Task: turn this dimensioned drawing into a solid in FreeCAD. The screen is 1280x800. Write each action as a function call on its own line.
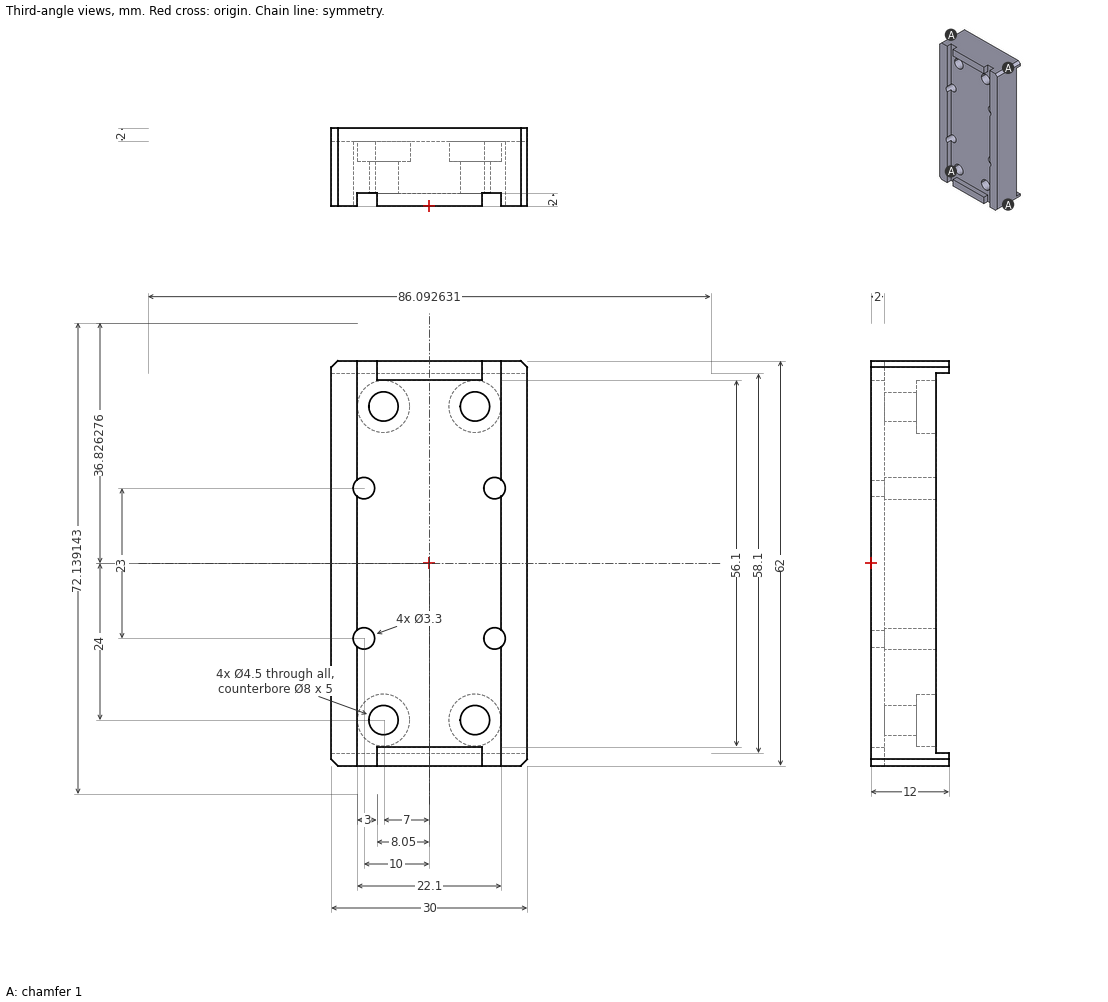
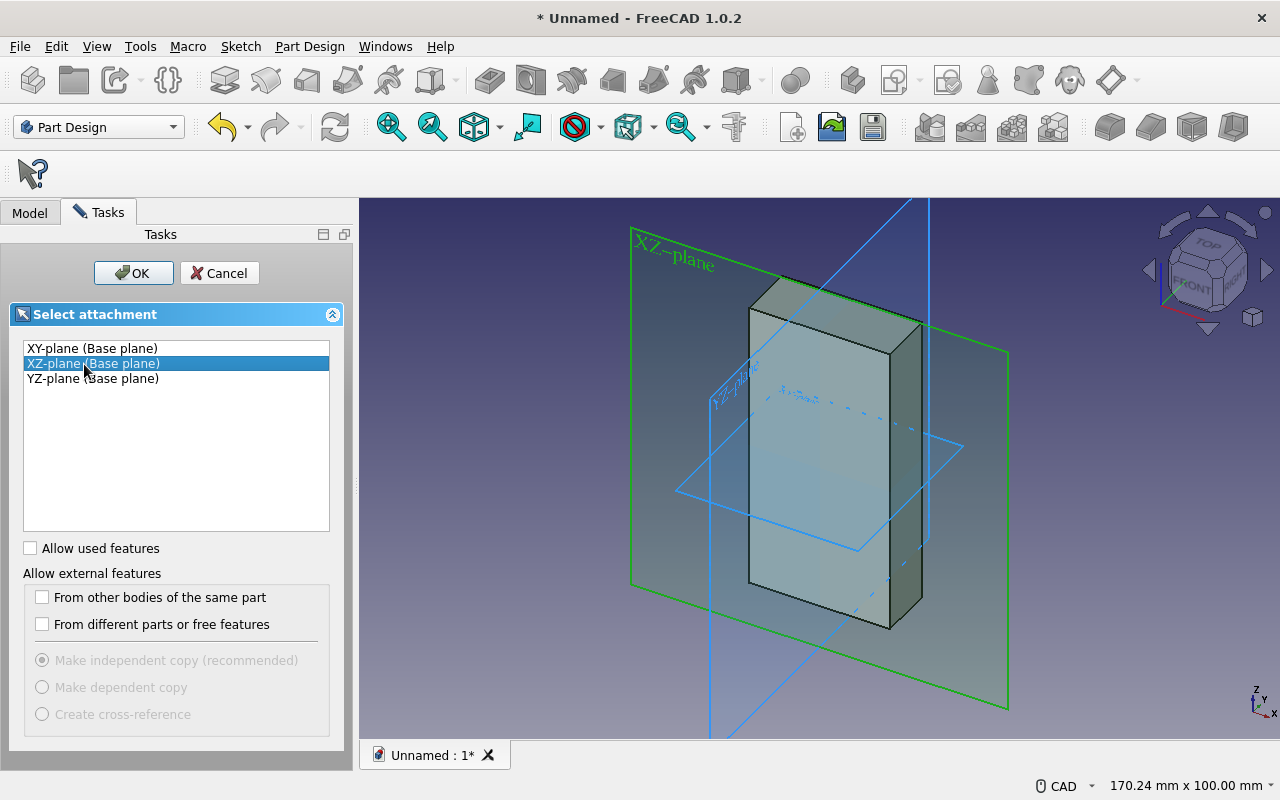
click(134, 273)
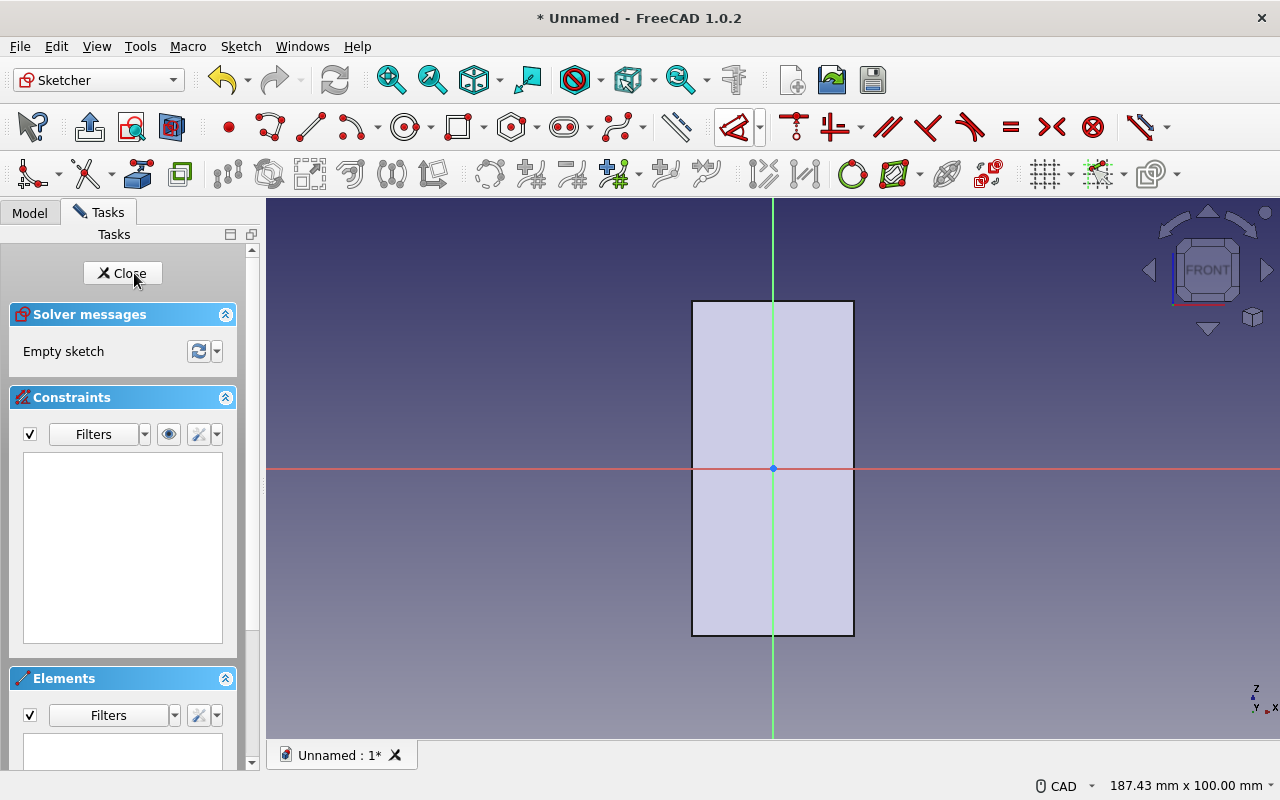
click(484, 128)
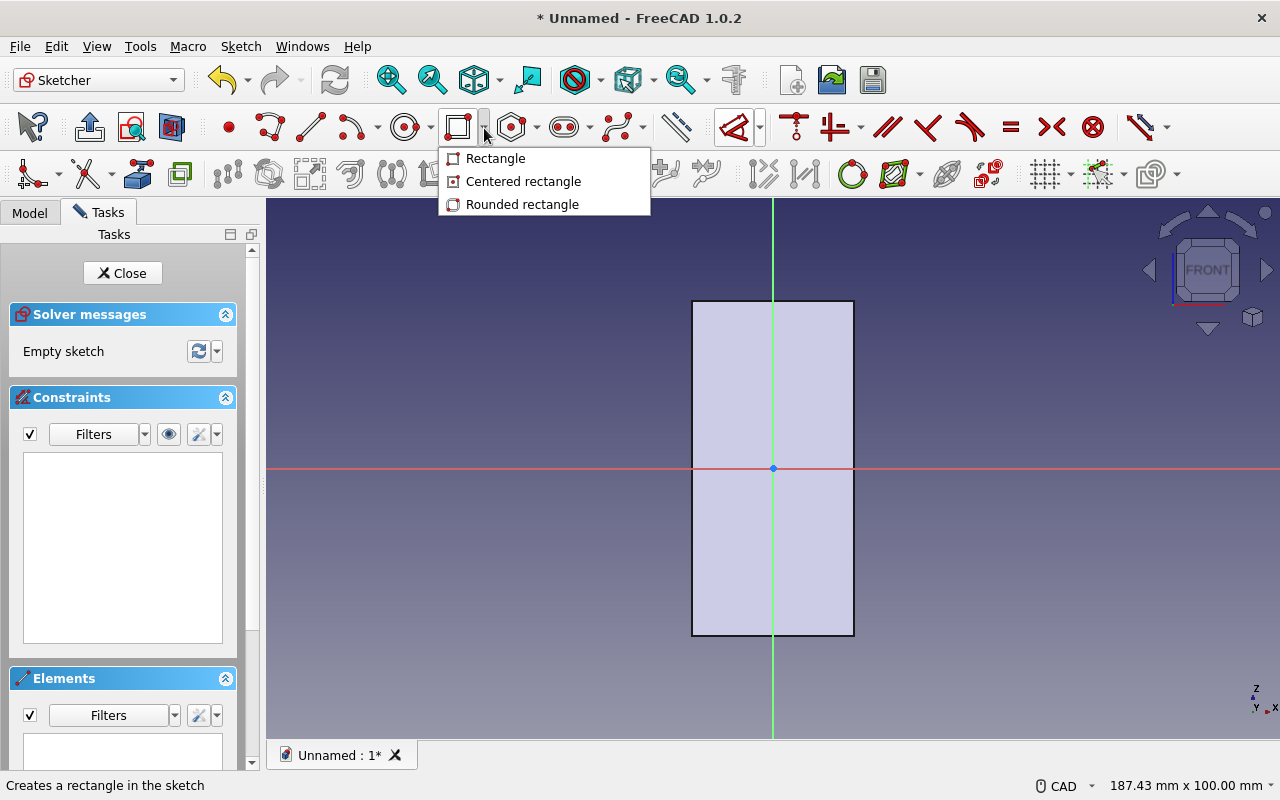
click(544, 182)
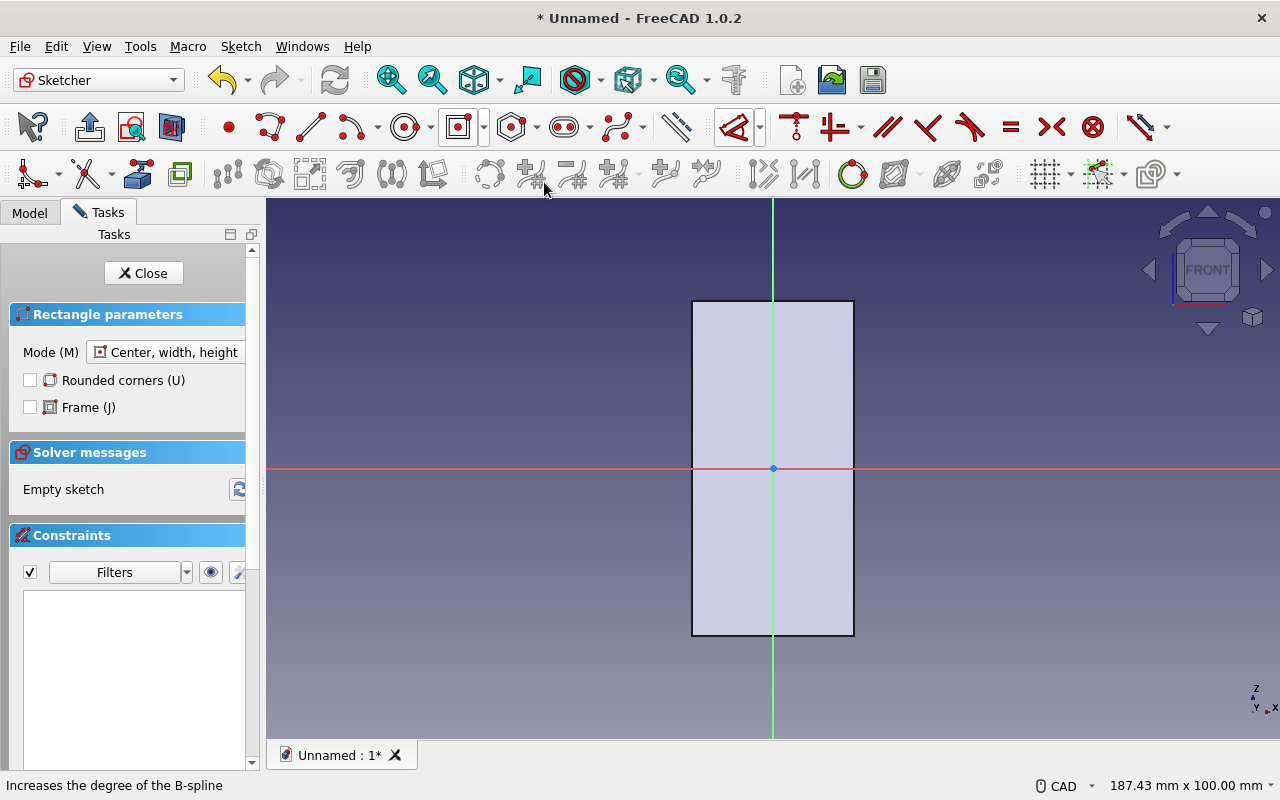
click(773, 468)
click(833, 317)
key(Escape)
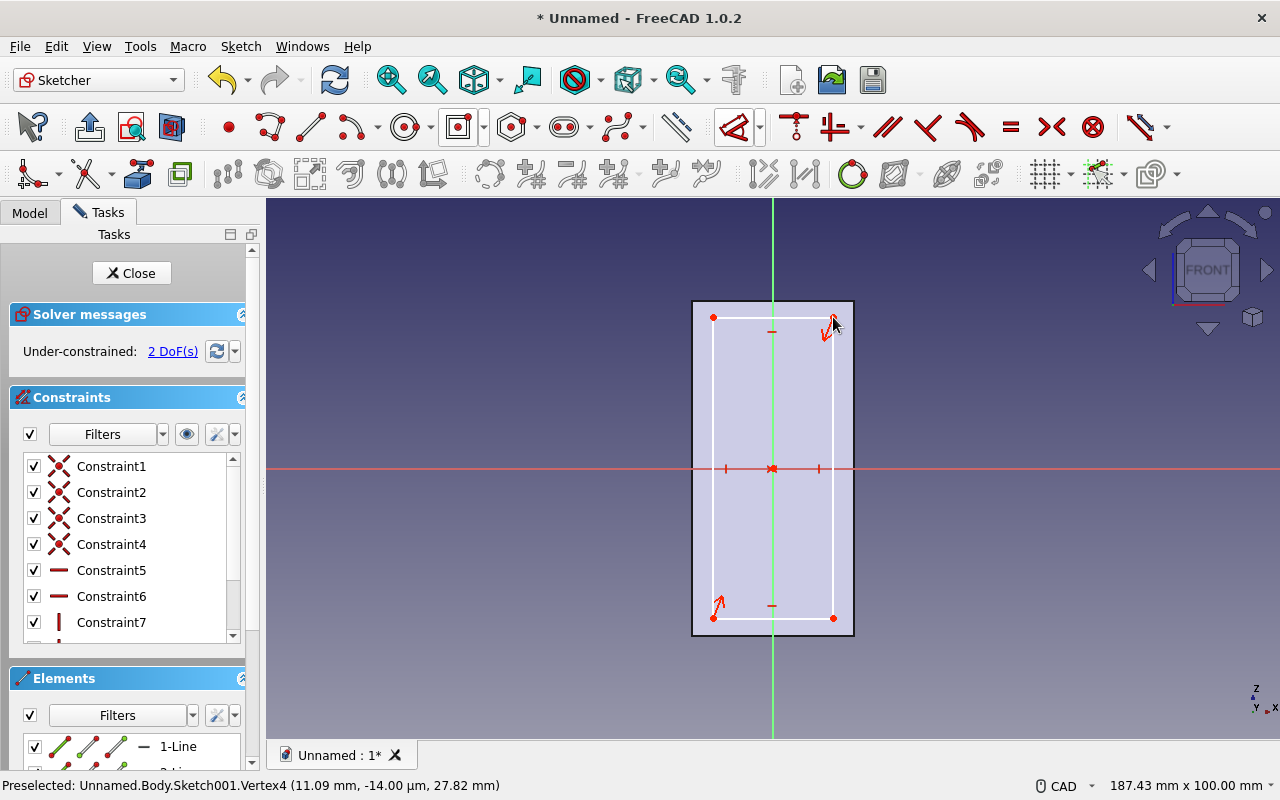
click(749, 619)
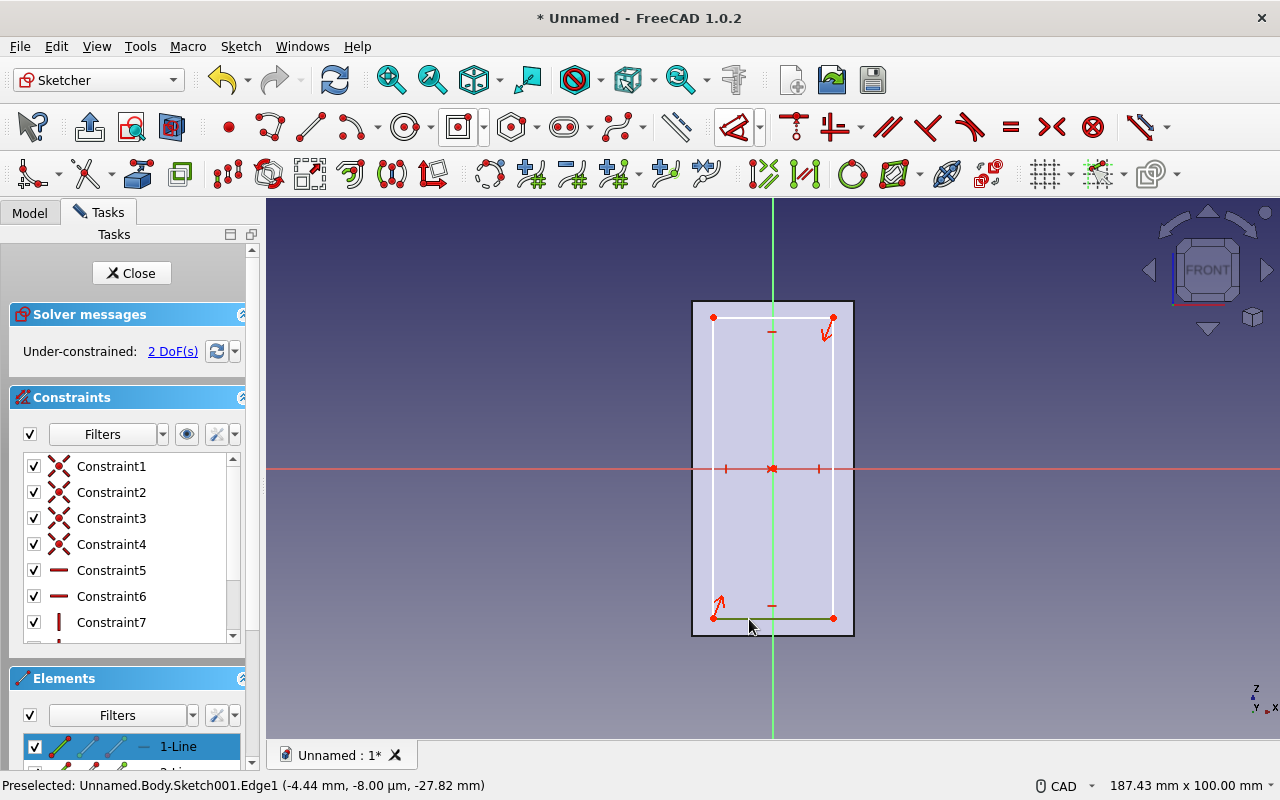
click(760, 128)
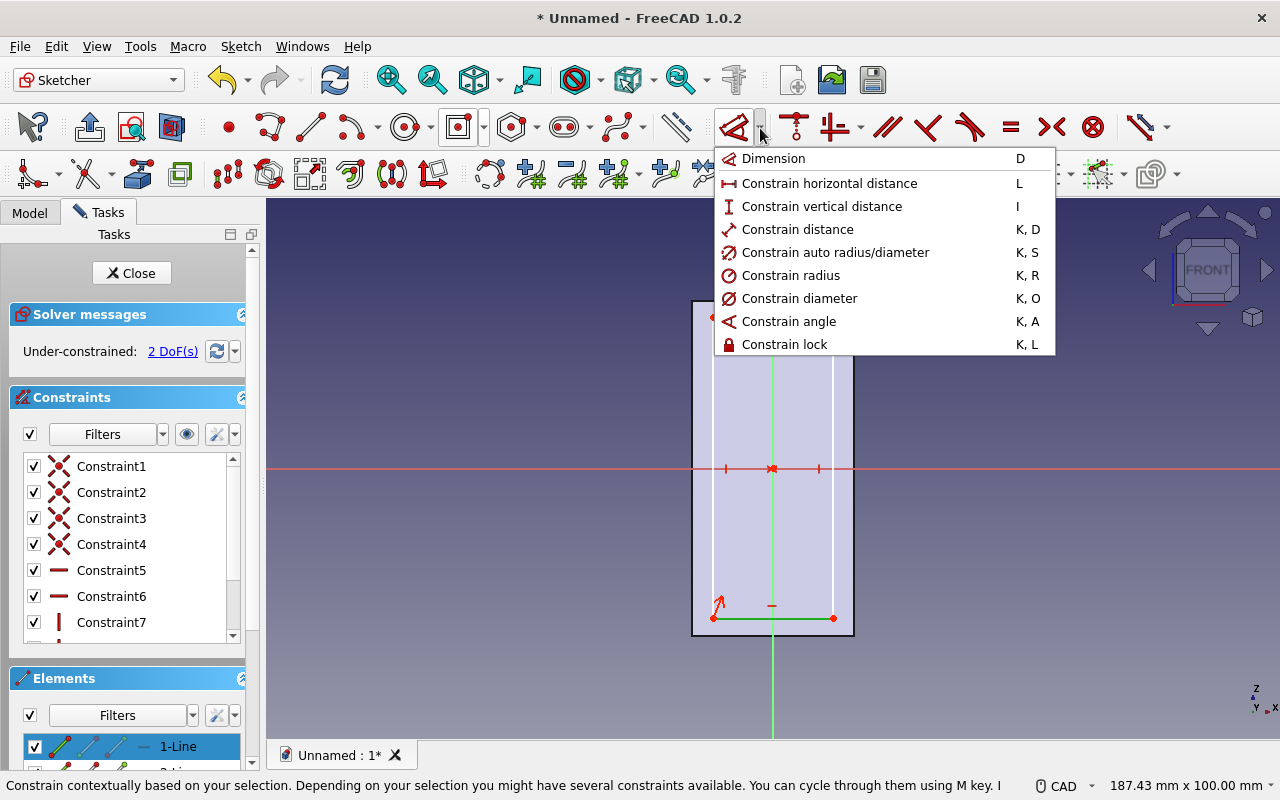
click(885, 184)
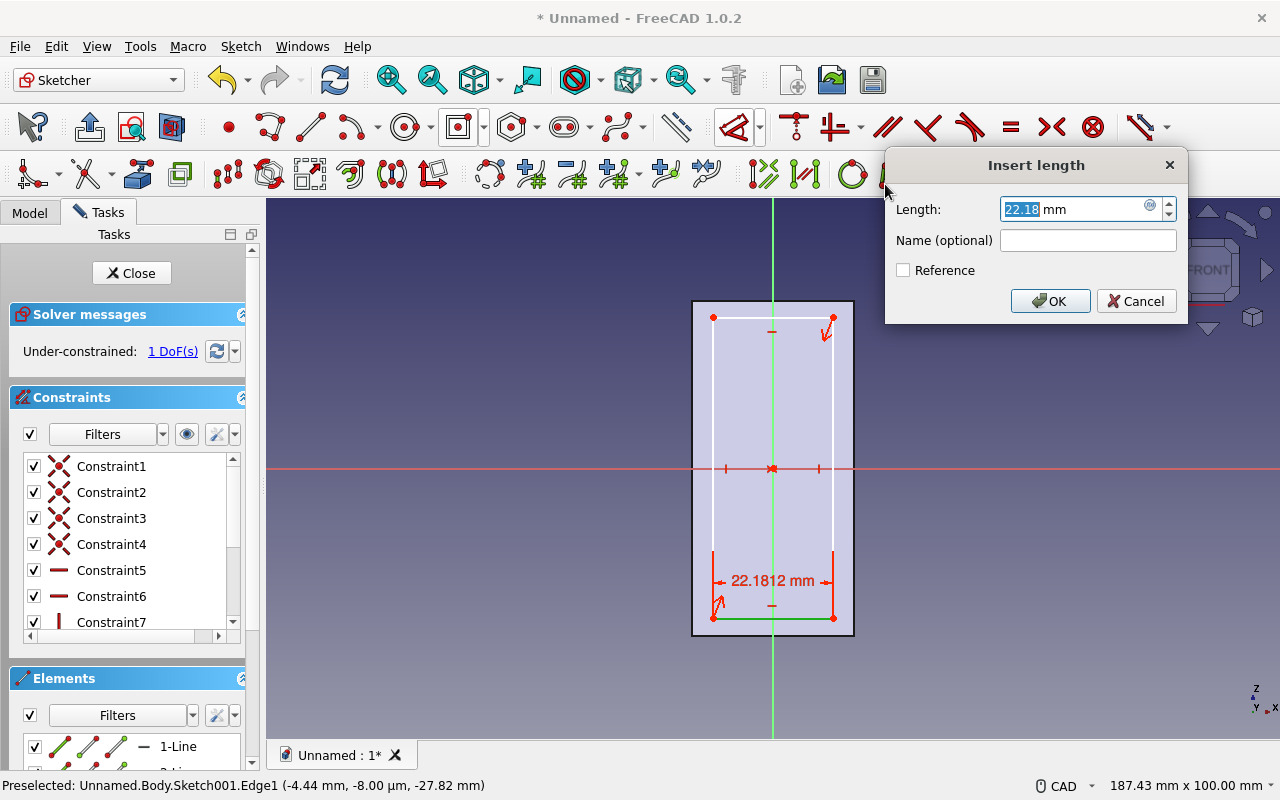
text(22.1)
key(Return)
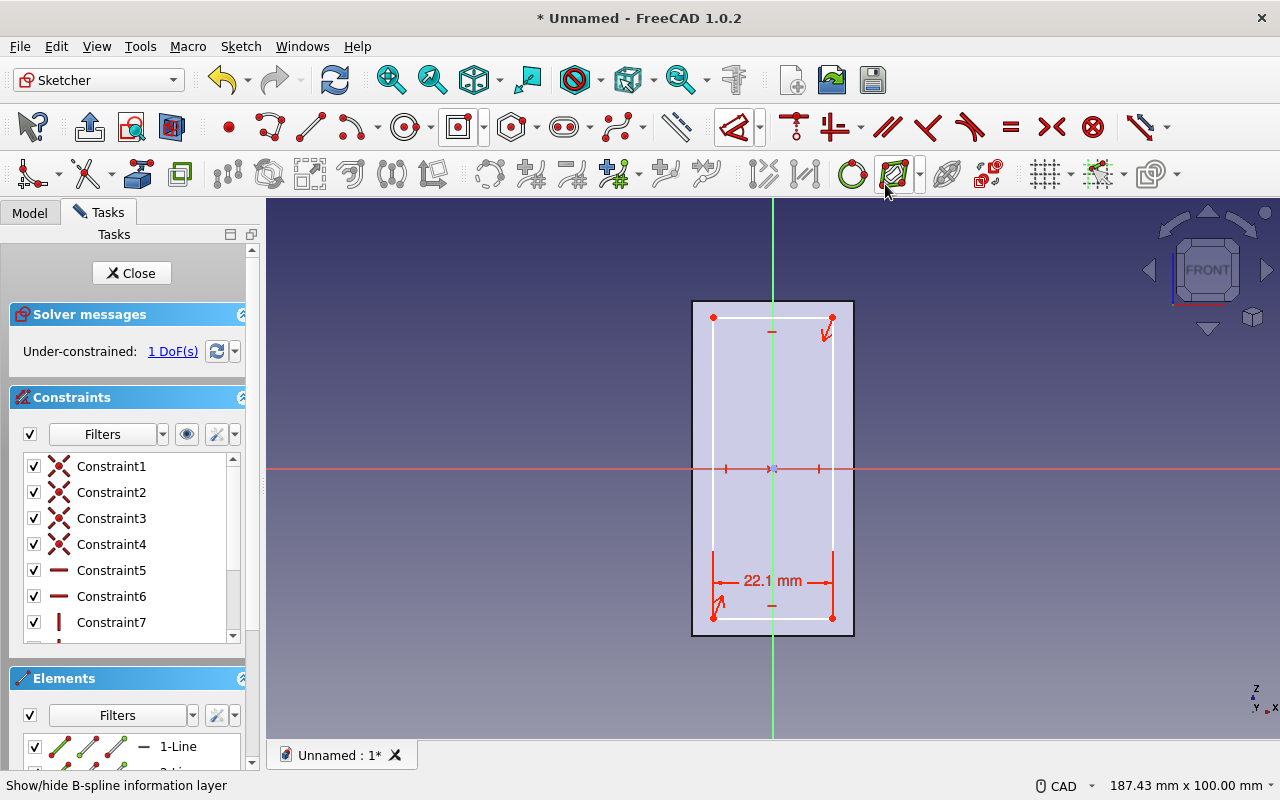
click(833, 529)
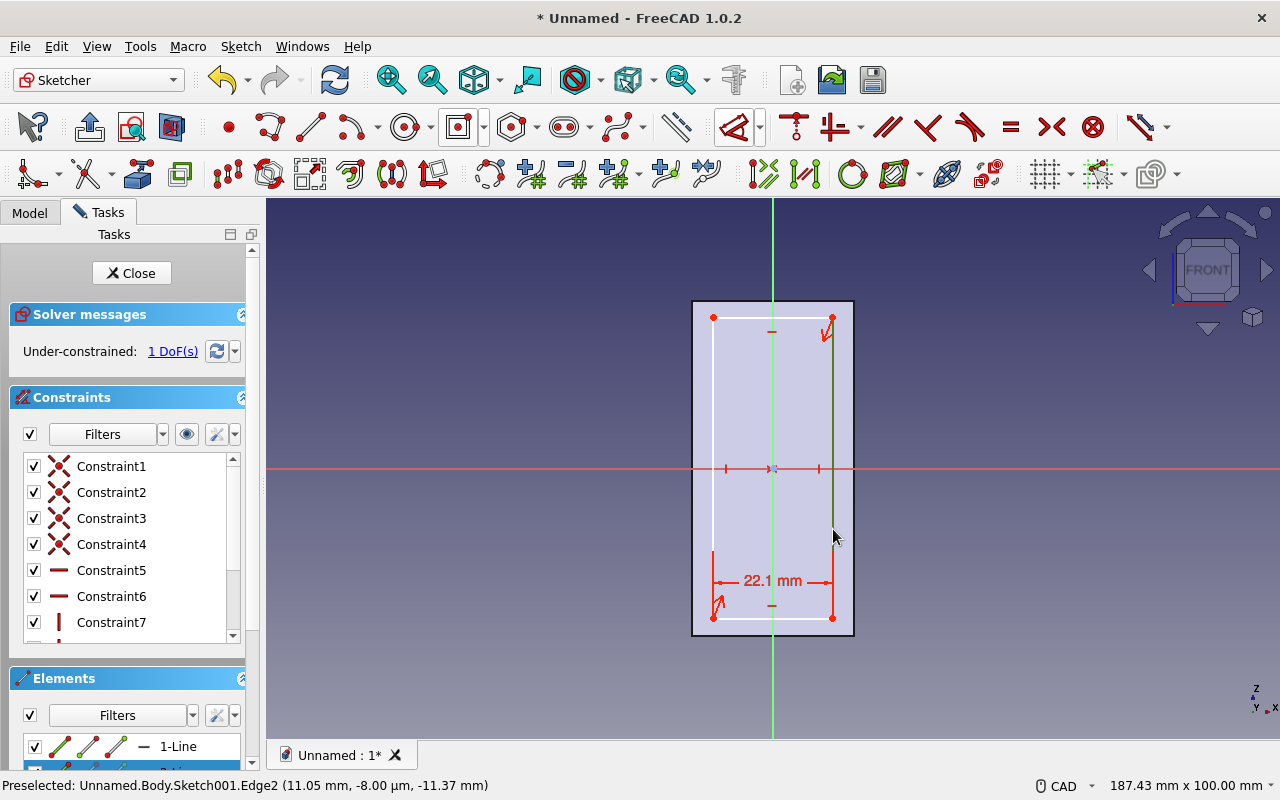
click(760, 128)